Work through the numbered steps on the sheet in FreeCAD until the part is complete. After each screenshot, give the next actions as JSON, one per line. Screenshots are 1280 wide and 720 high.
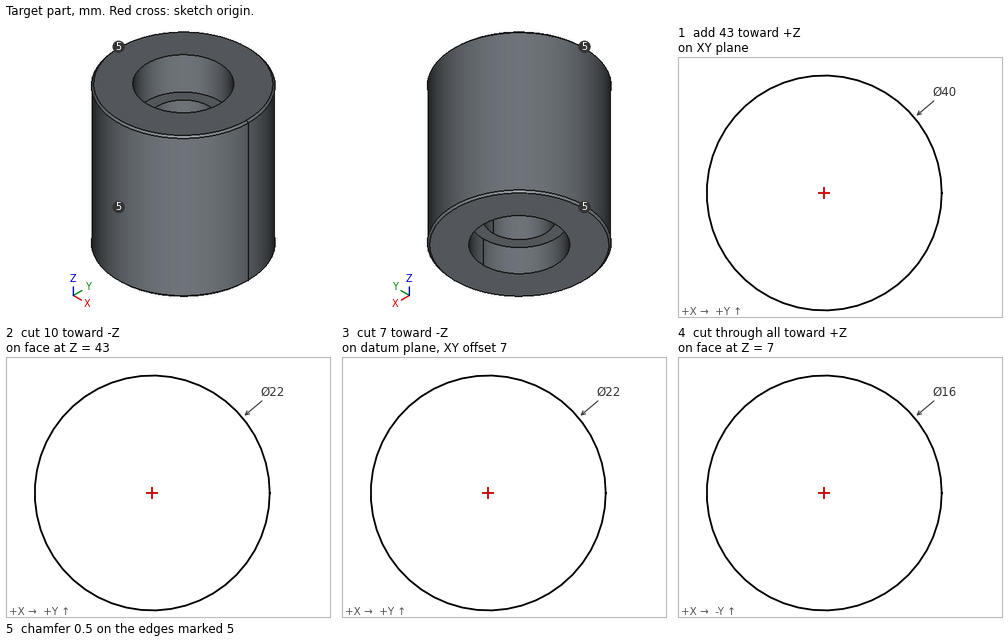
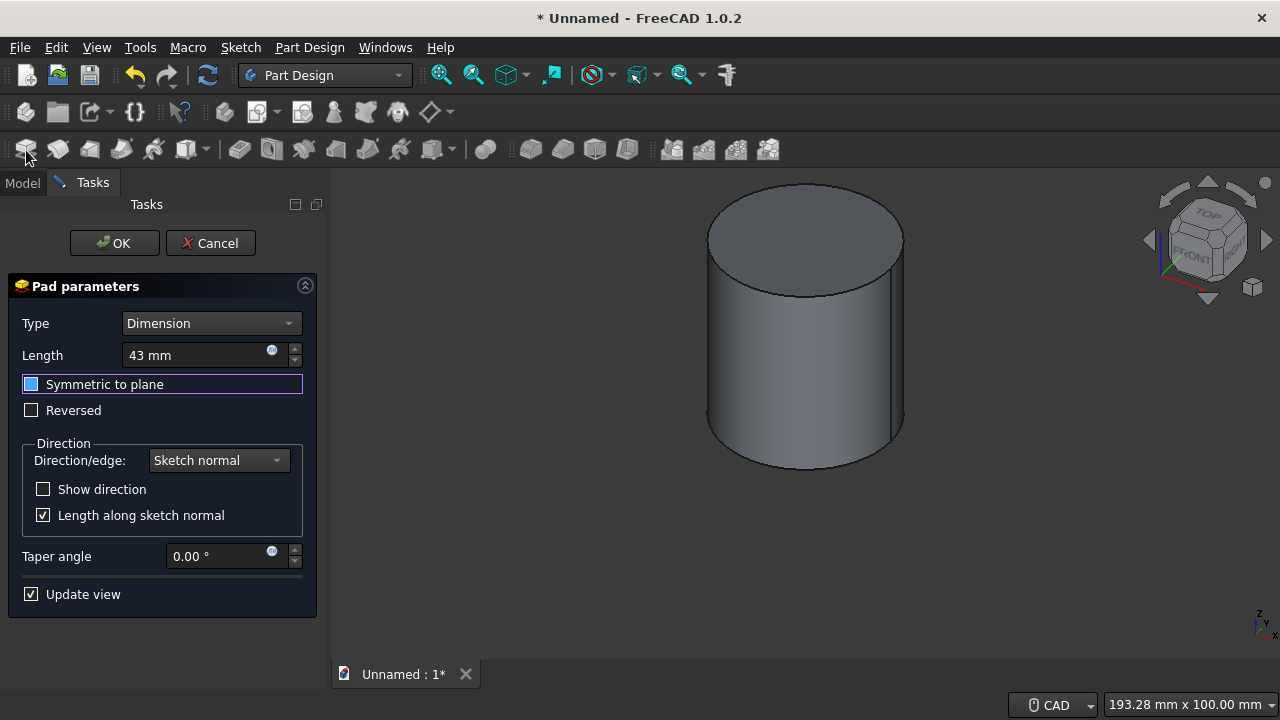
{"action": "left_click", "coordinate": [115, 243]}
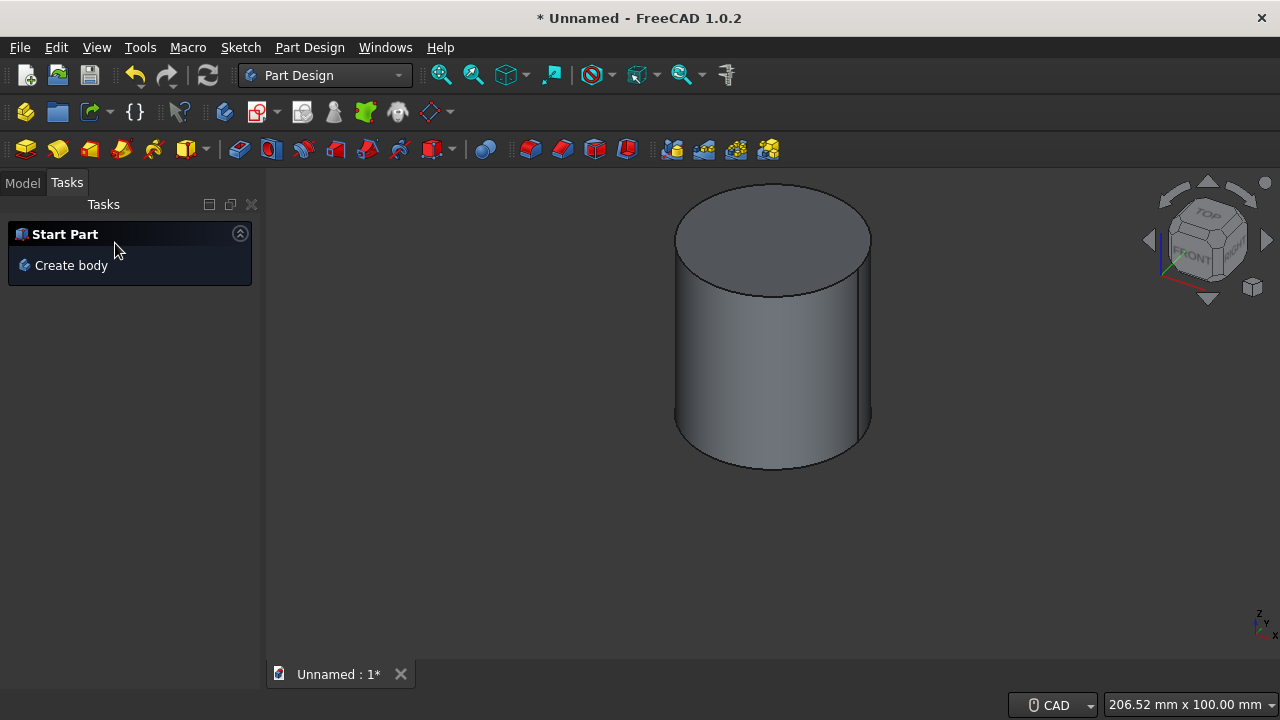
{"action": "left_click", "coordinate": [442, 76]}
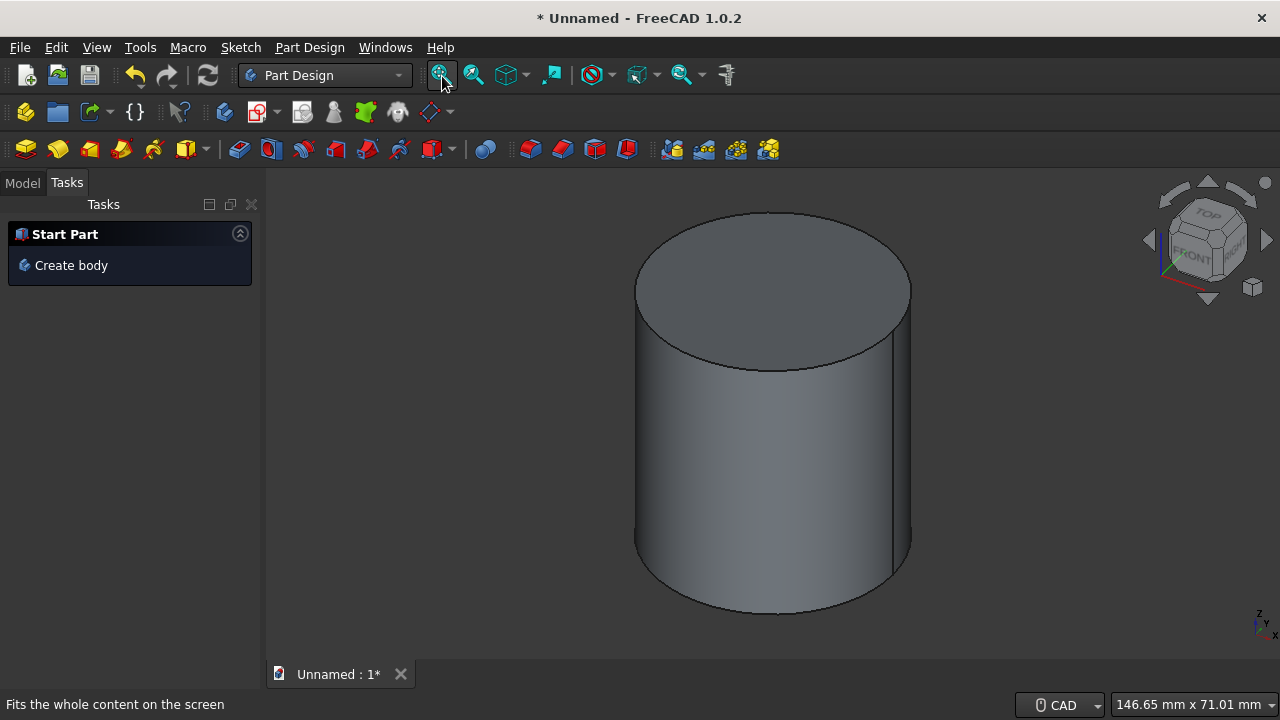
{"action": "left_click", "coordinate": [773, 291]}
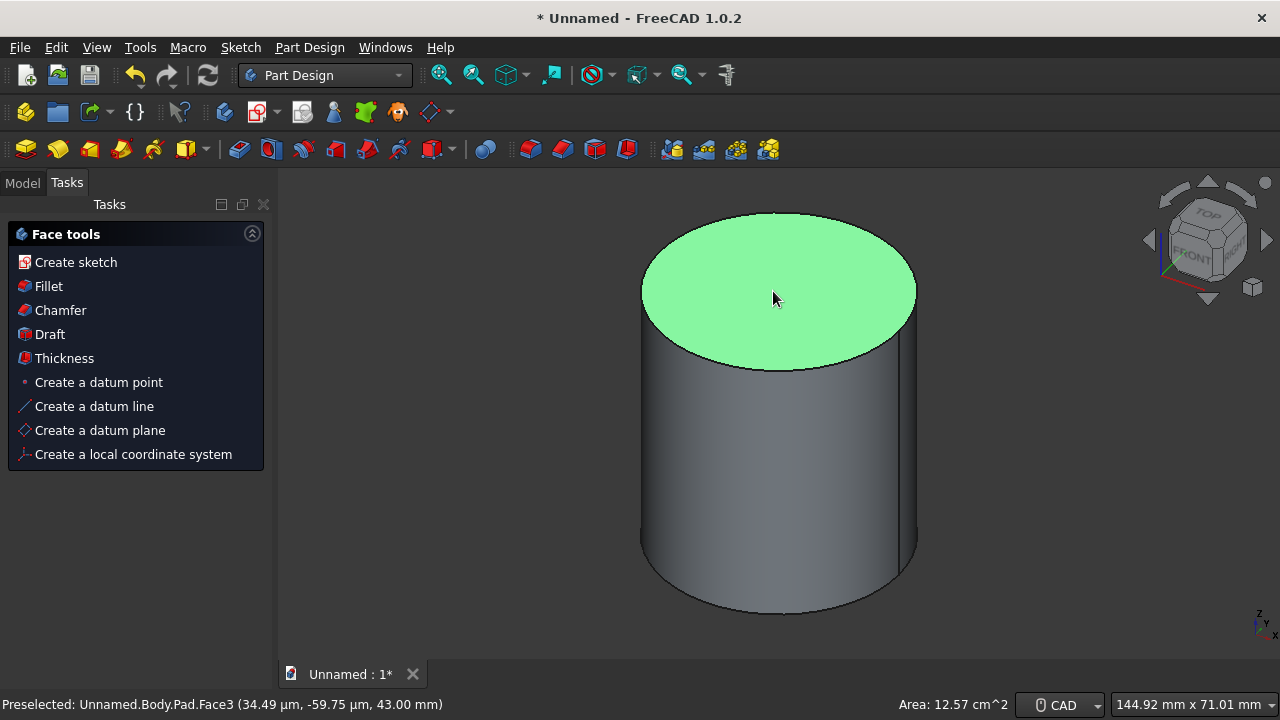
{"action": "left_click", "coordinate": [258, 112]}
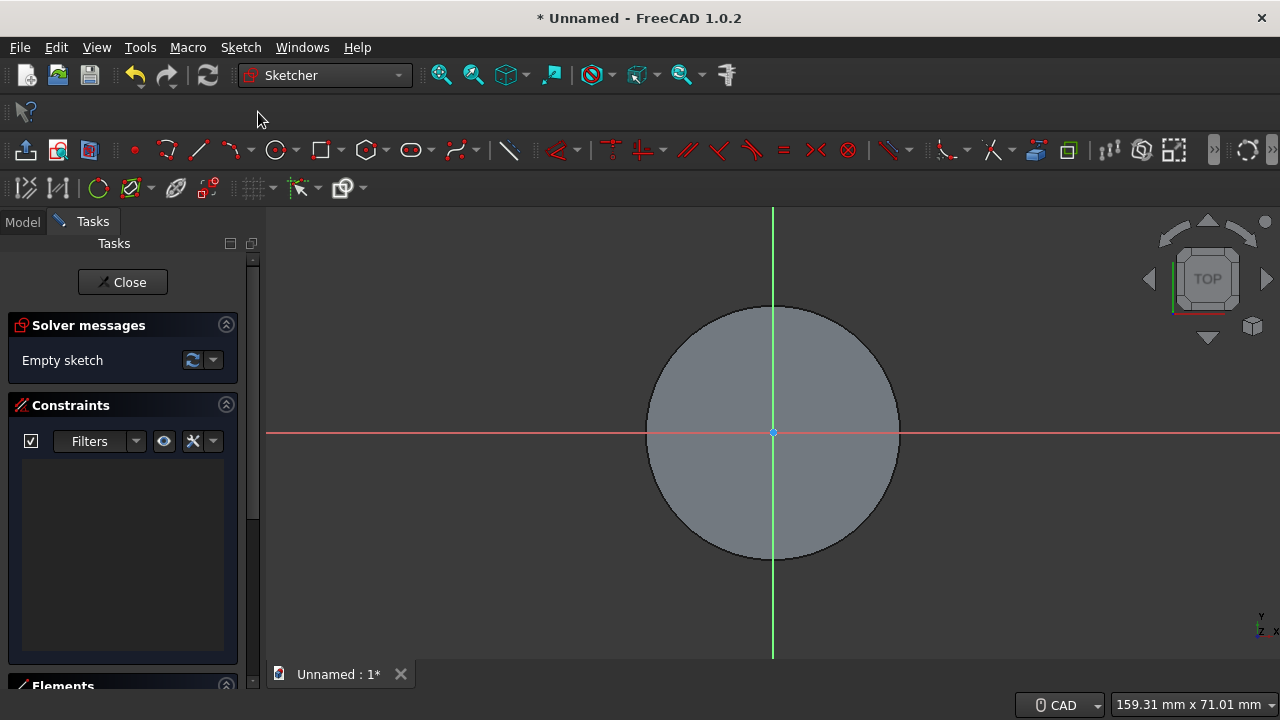
{"action": "scroll", "coordinate": [856, 433], "scroll_direction": "up", "scroll_amount": 3}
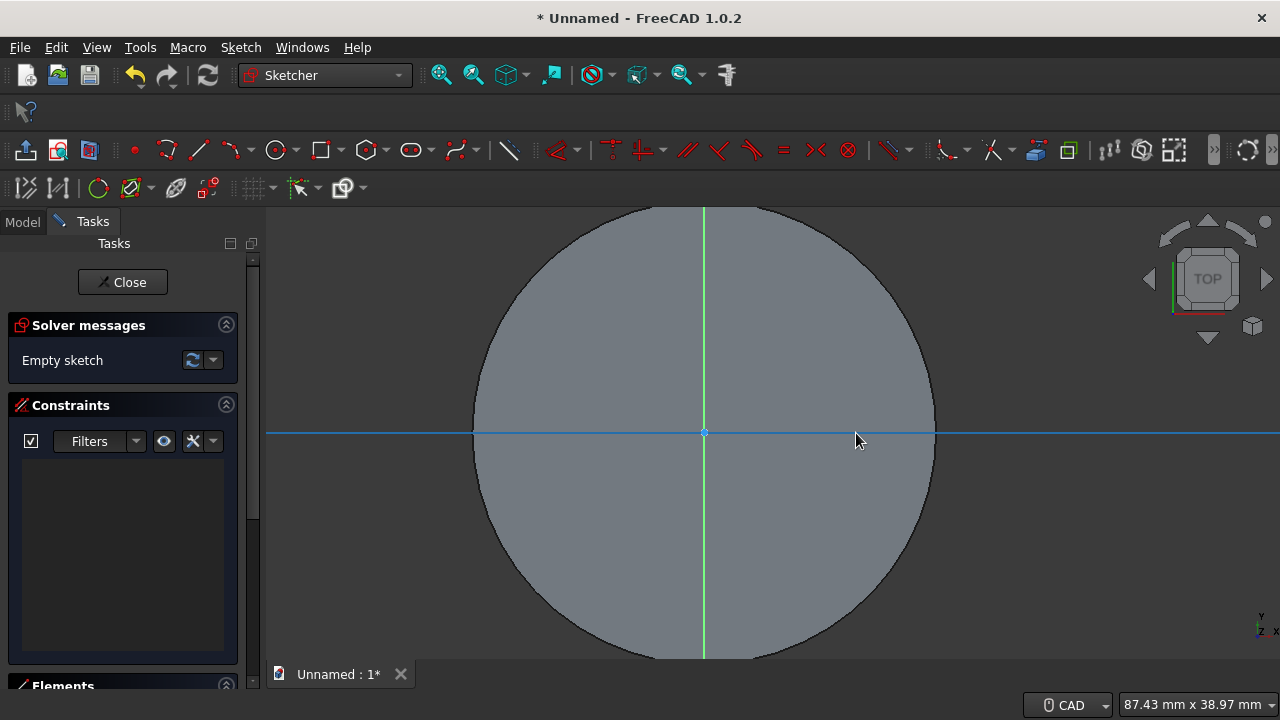
{"action": "left_click", "coordinate": [276, 150]}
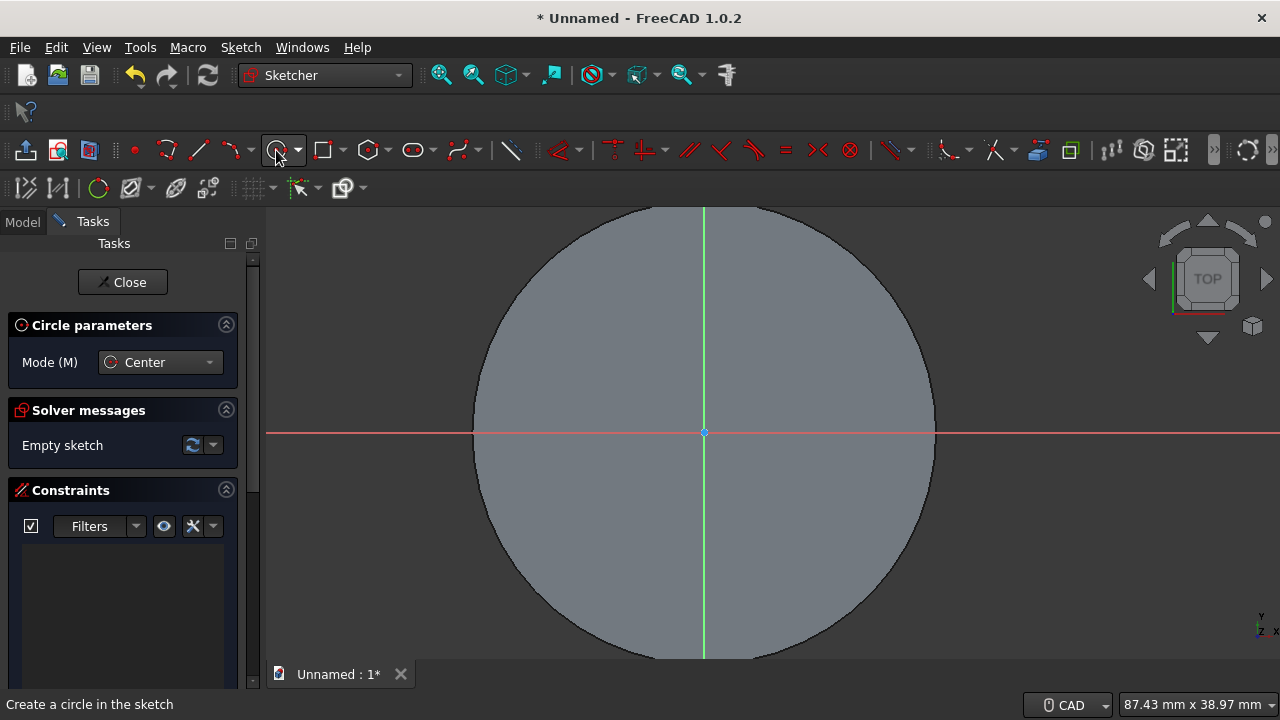
{"action": "left_click", "coordinate": [704, 433]}
{"action": "mouse_move", "coordinate": [794, 342]}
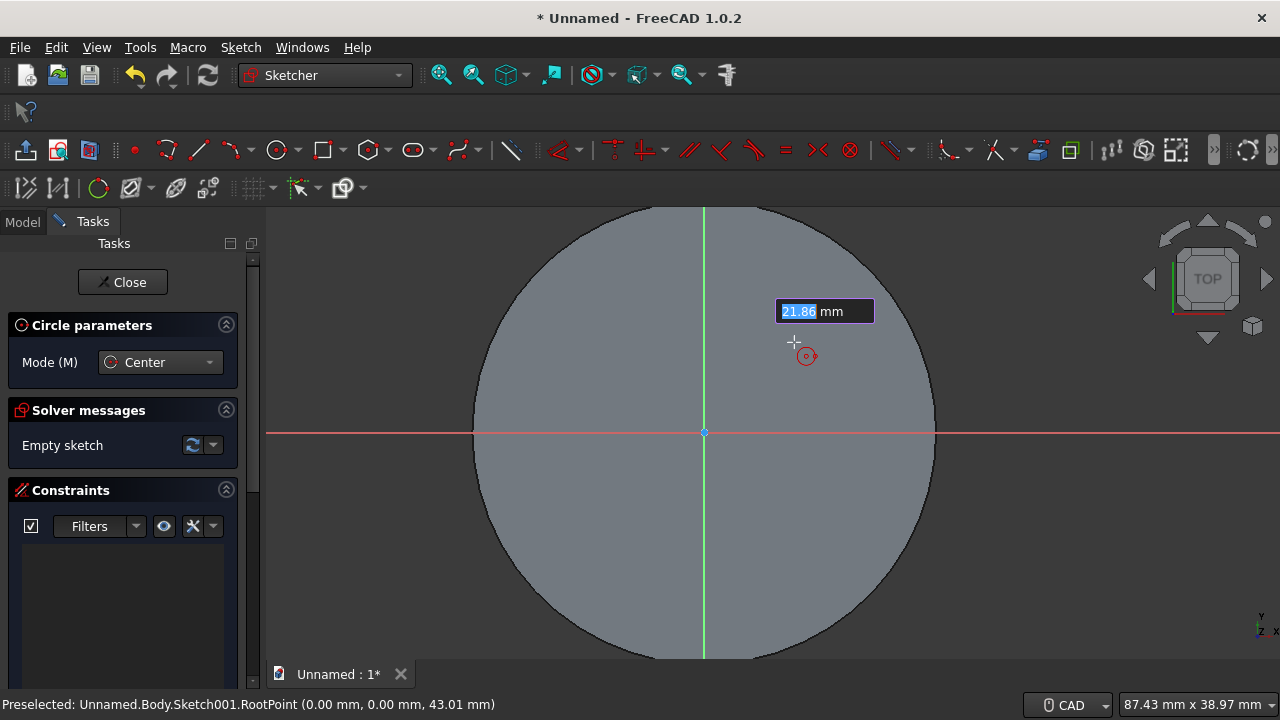
{"action": "type", "text": "22"}
{"action": "key", "text": "Return"}
{"action": "key", "text": "Escape"}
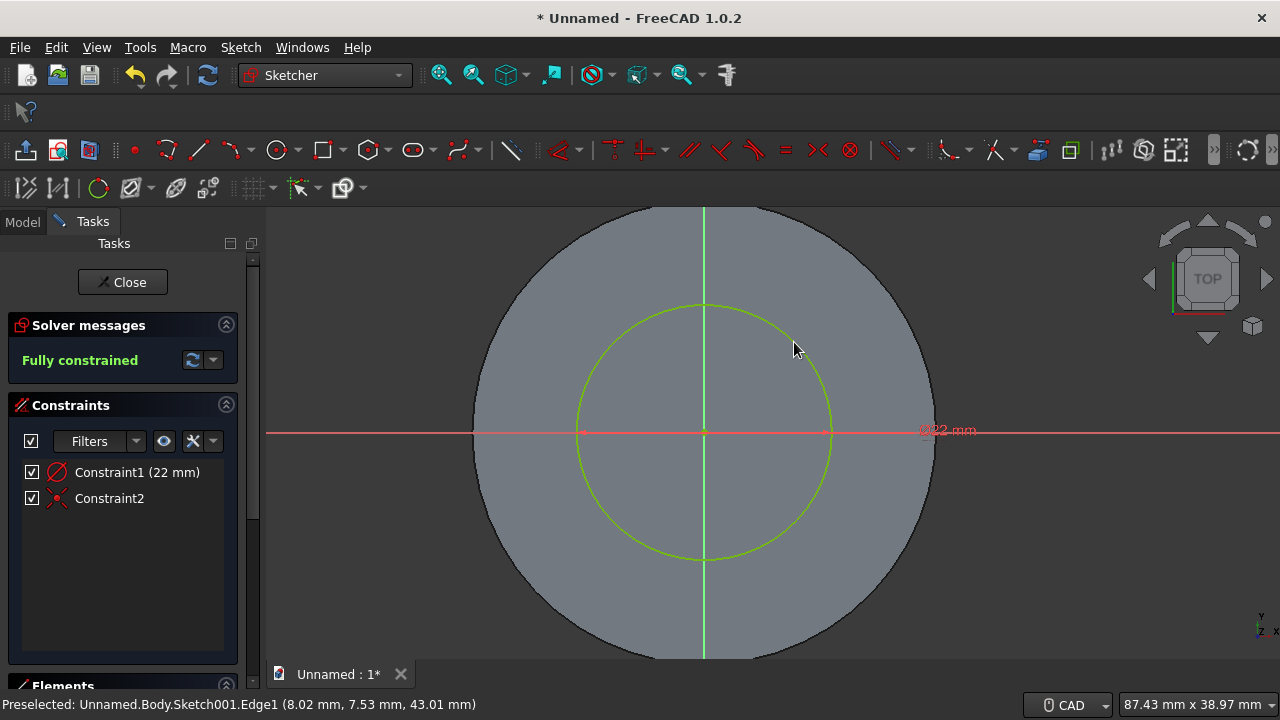
{"action": "left_click", "coordinate": [123, 282]}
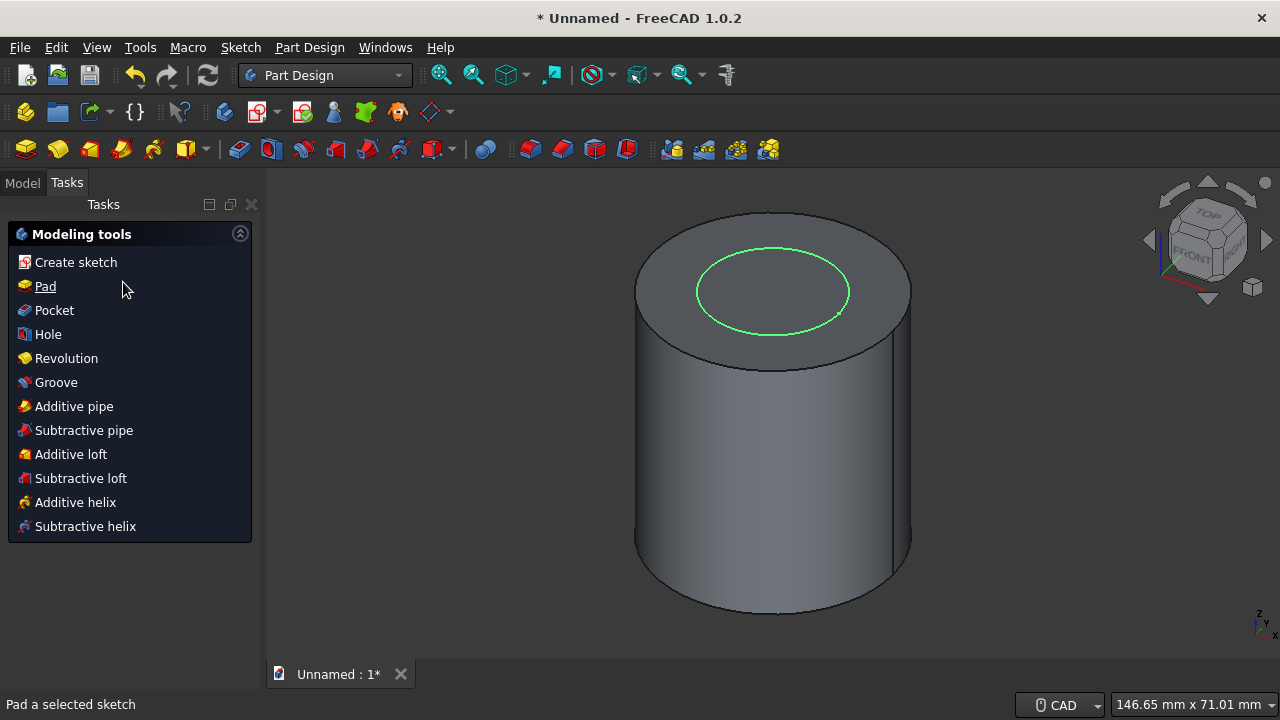
{"action": "left_click", "coordinate": [240, 150]}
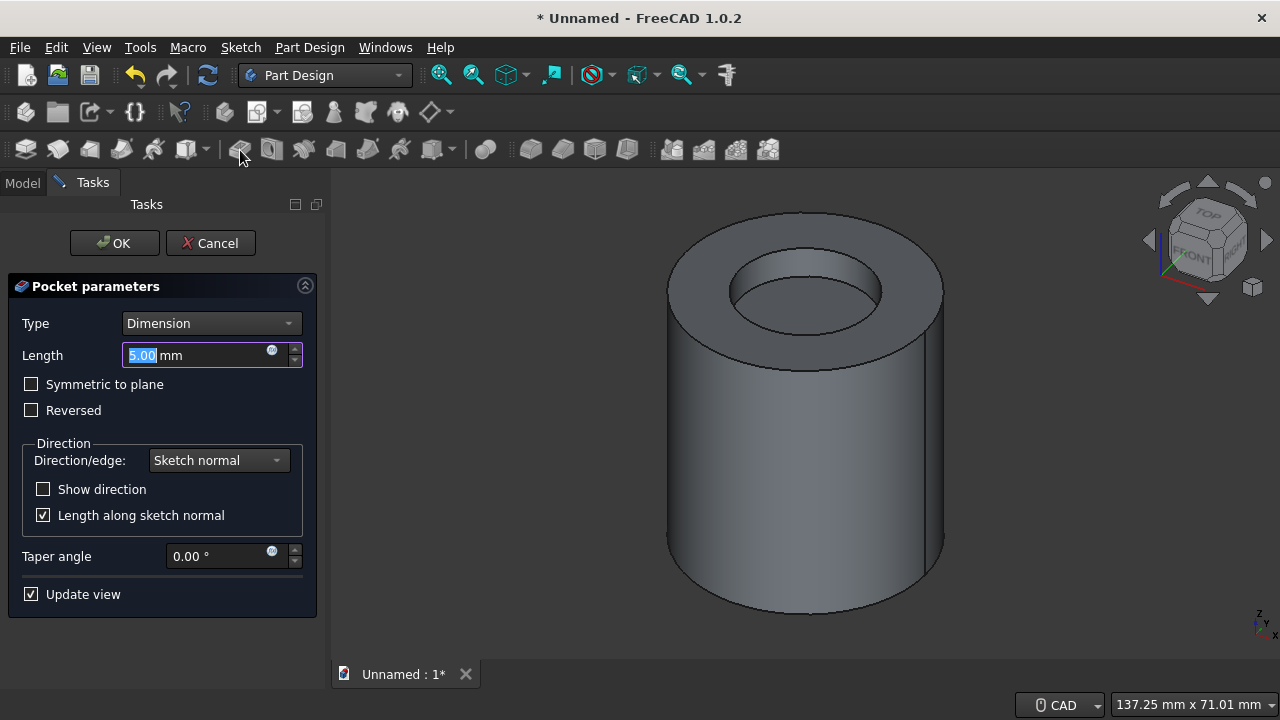
{"action": "type", "text": "10"}
{"action": "key", "text": "Tab"}